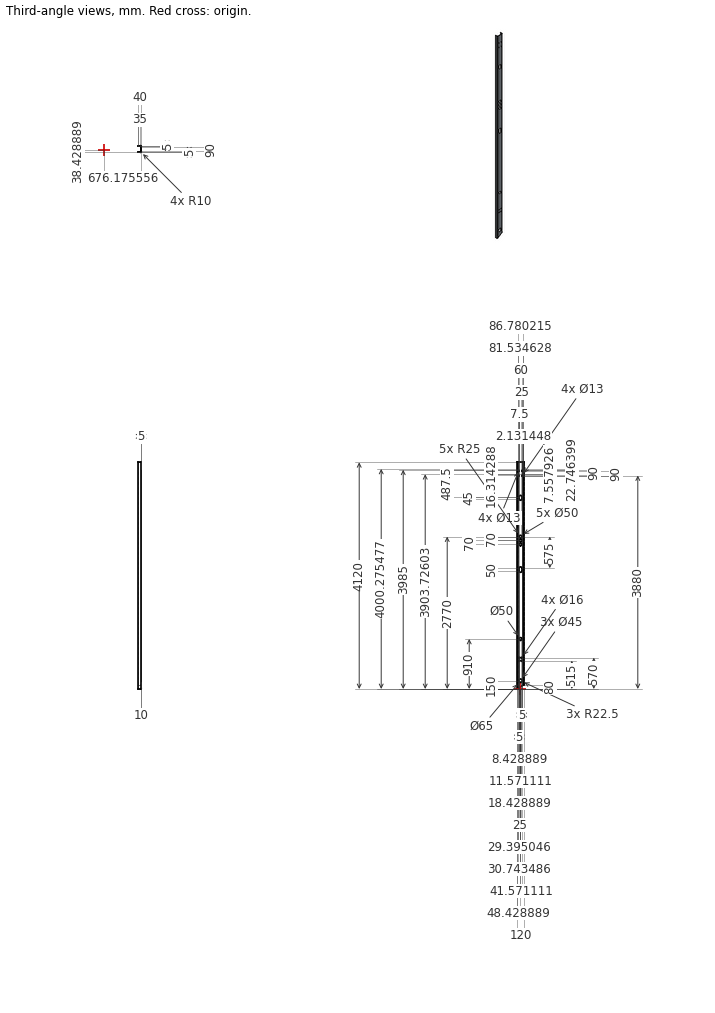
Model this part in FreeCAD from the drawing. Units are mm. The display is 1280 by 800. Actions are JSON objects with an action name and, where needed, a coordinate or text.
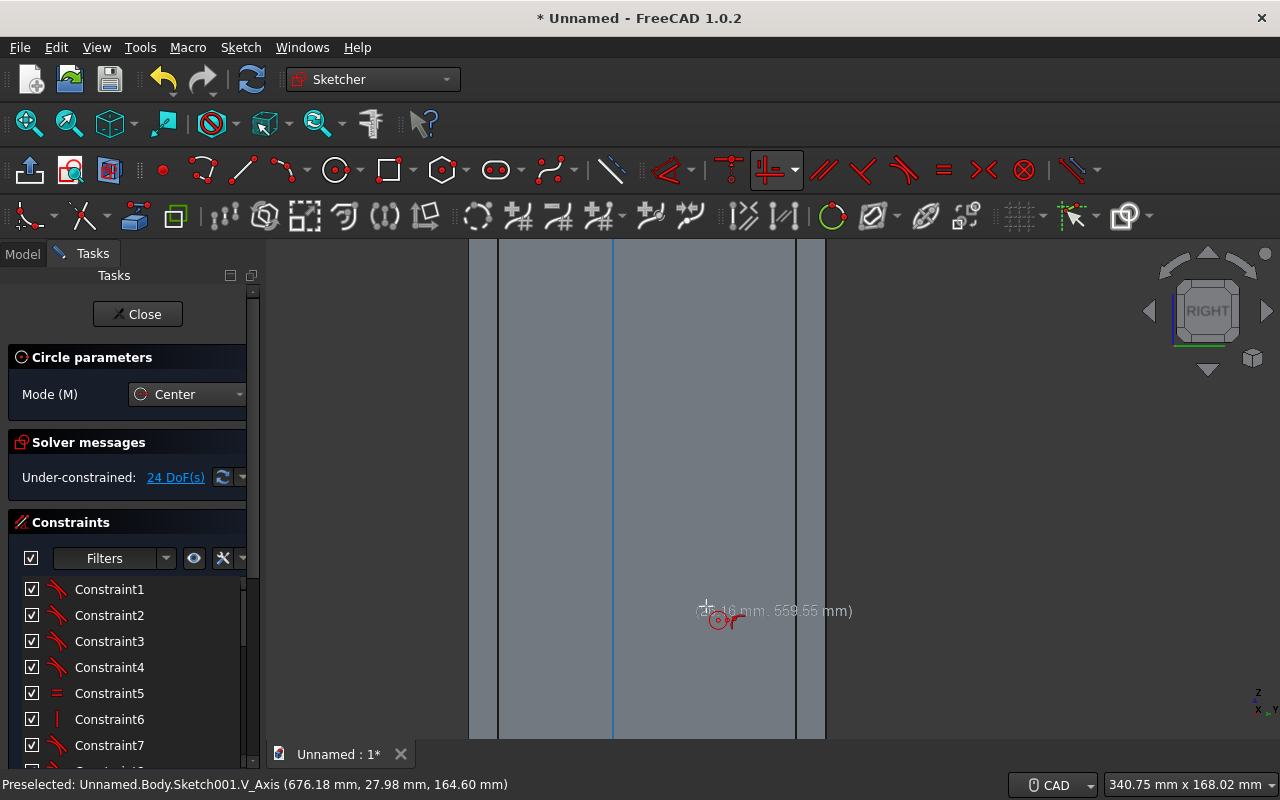
{"action": "scroll", "coordinate": [706, 605], "scroll_direction": "down", "scroll_amount": 18}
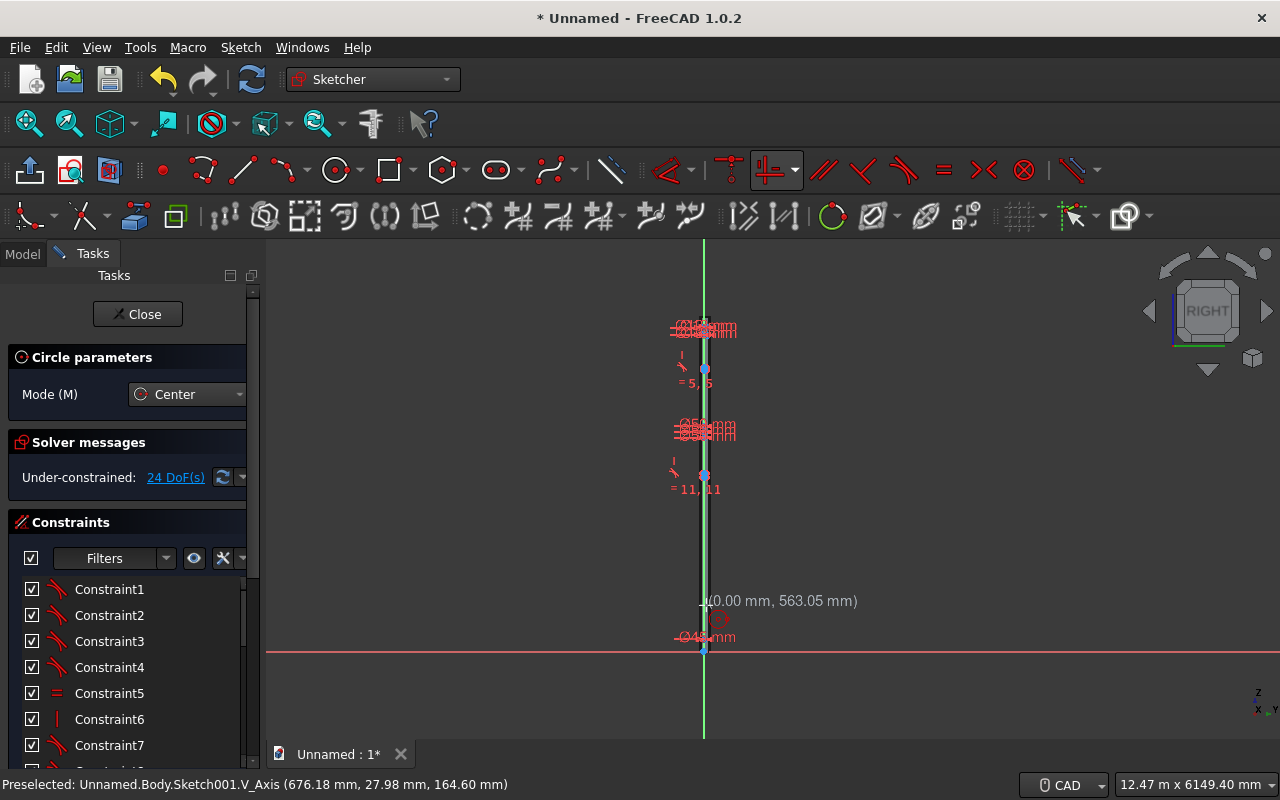
{"action": "scroll", "coordinate": [706, 605], "scroll_direction": "up", "scroll_amount": 10}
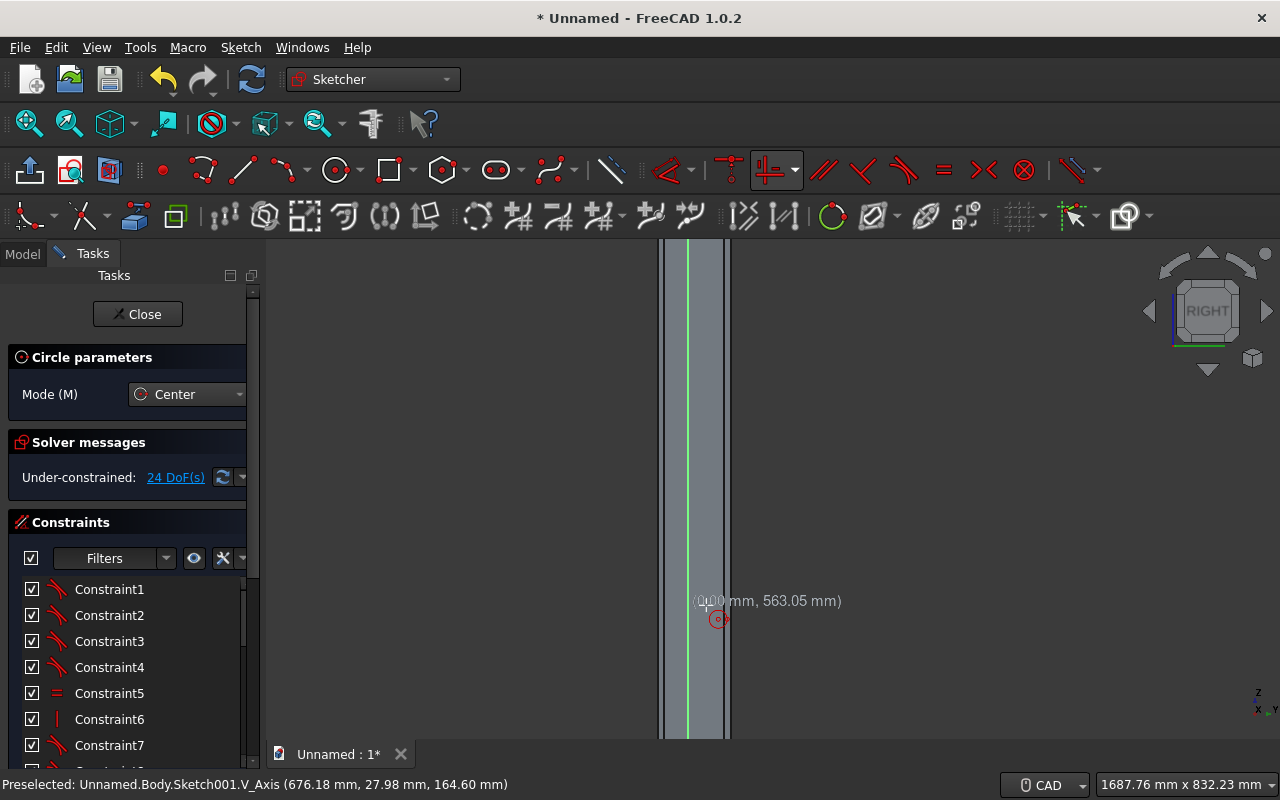
{"action": "left_click", "coordinate": [706, 602]}
{"action": "mouse_move", "coordinate": [710, 598]}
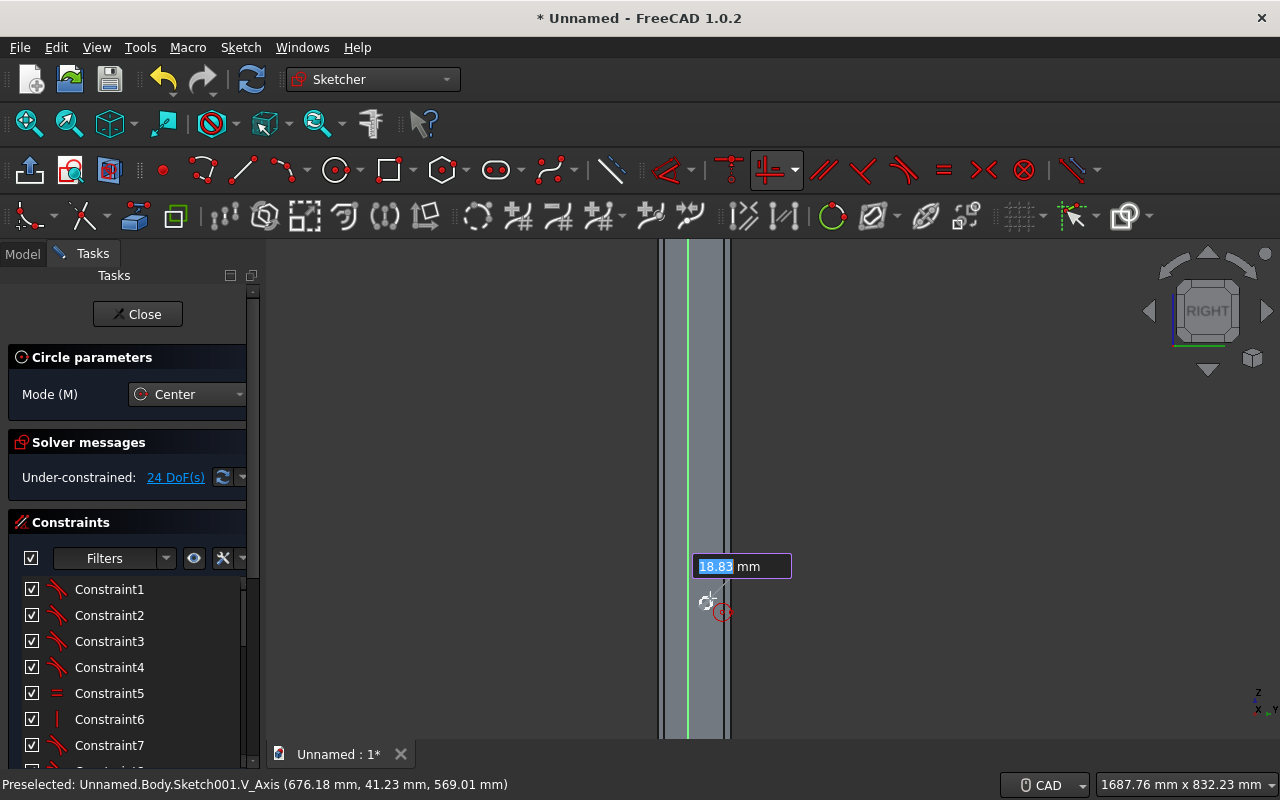
{"action": "type", "text": "16"}
{"action": "key", "text": "Return"}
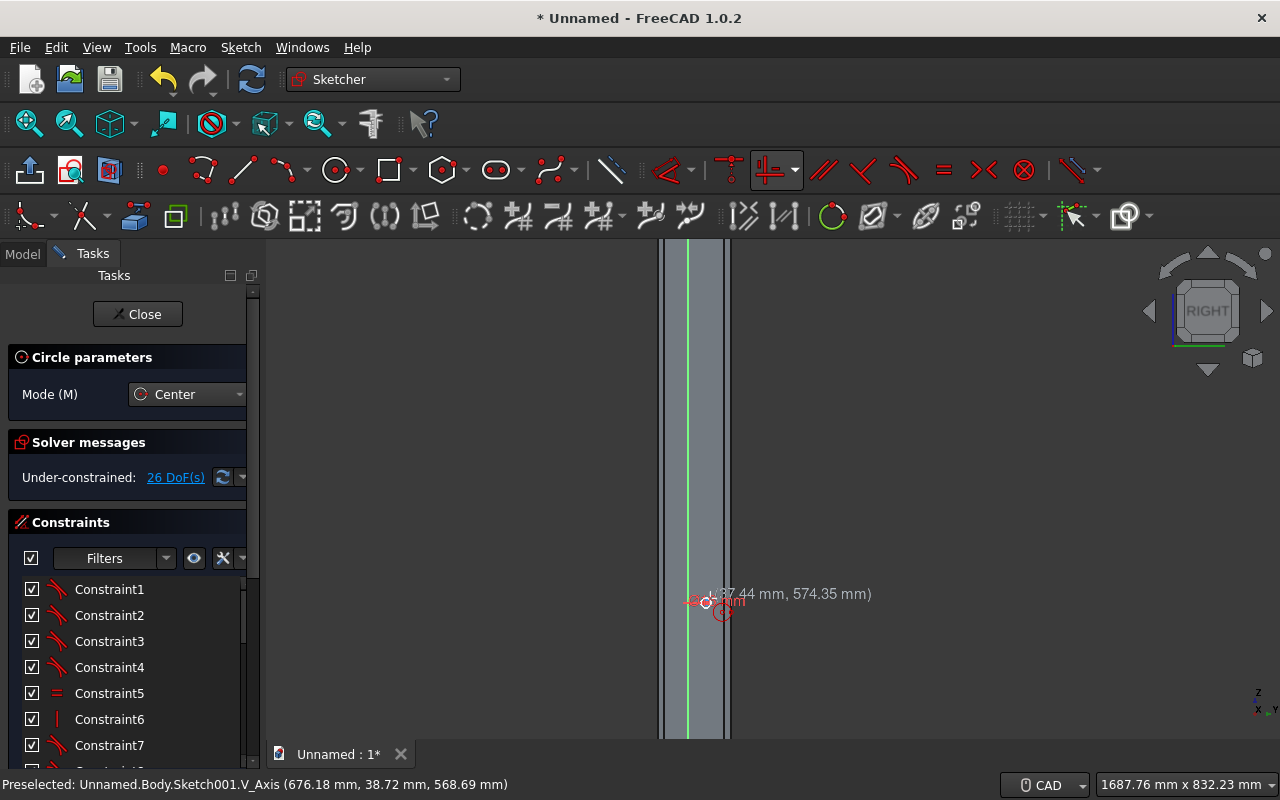
{"action": "scroll", "coordinate": [706, 635], "scroll_direction": "up", "scroll_amount": 8}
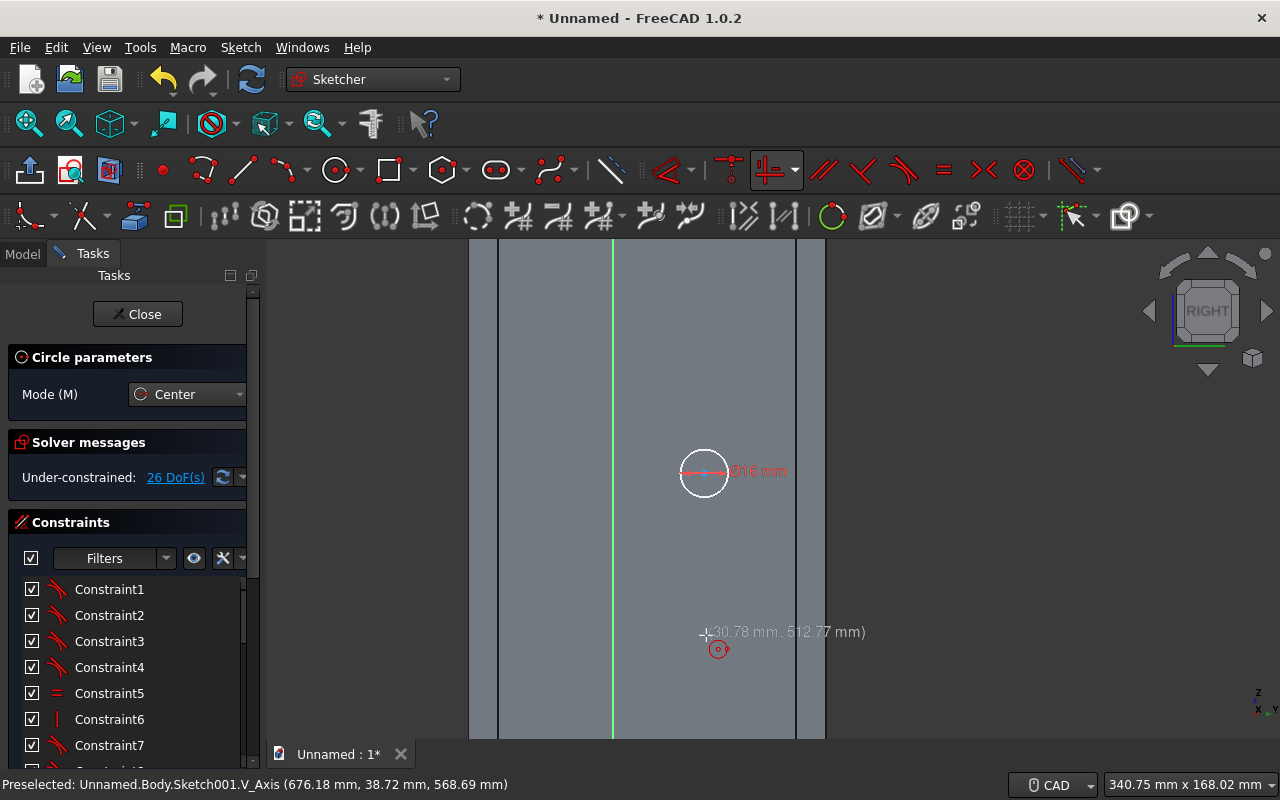
{"action": "scroll", "coordinate": [706, 609], "scroll_direction": "down", "scroll_amount": 18}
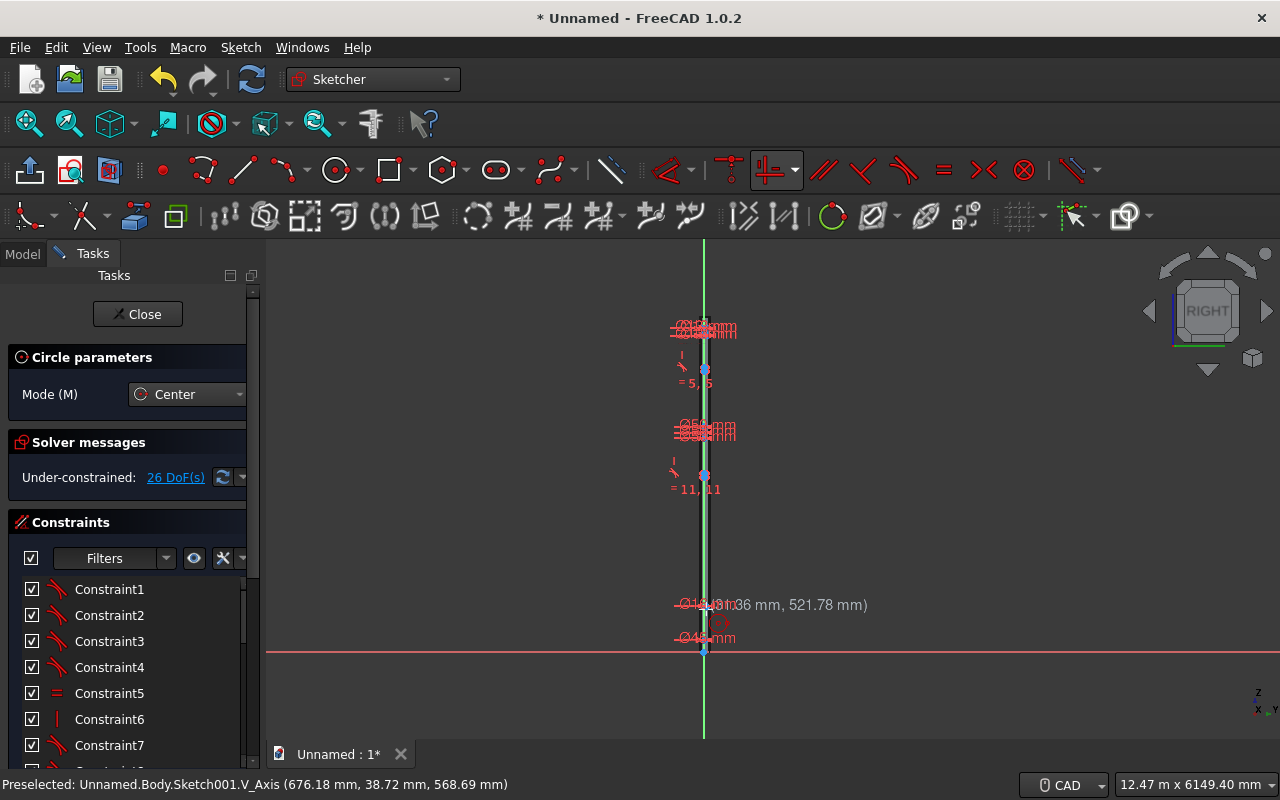
{"action": "scroll", "coordinate": [706, 610], "scroll_direction": "up", "scroll_amount": 10}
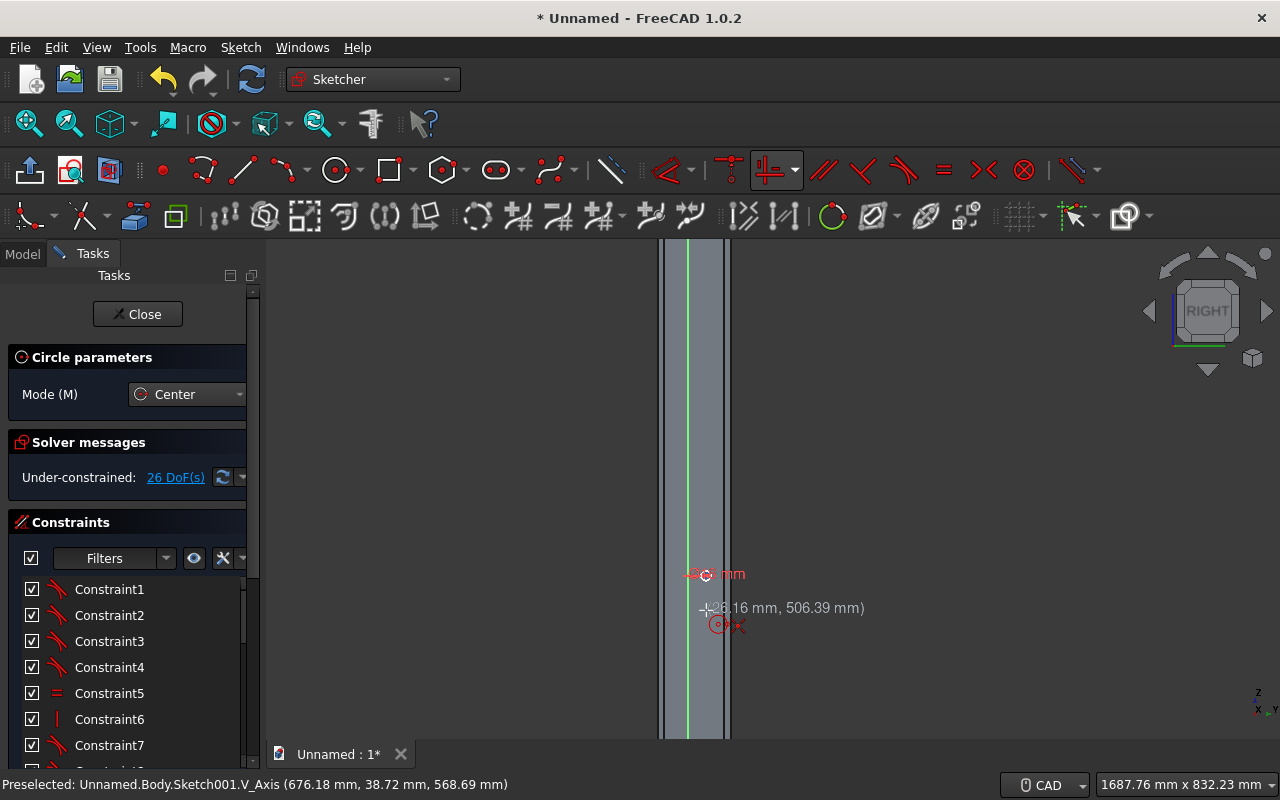
{"action": "left_click", "coordinate": [706, 607]}
{"action": "mouse_move", "coordinate": [710, 604]}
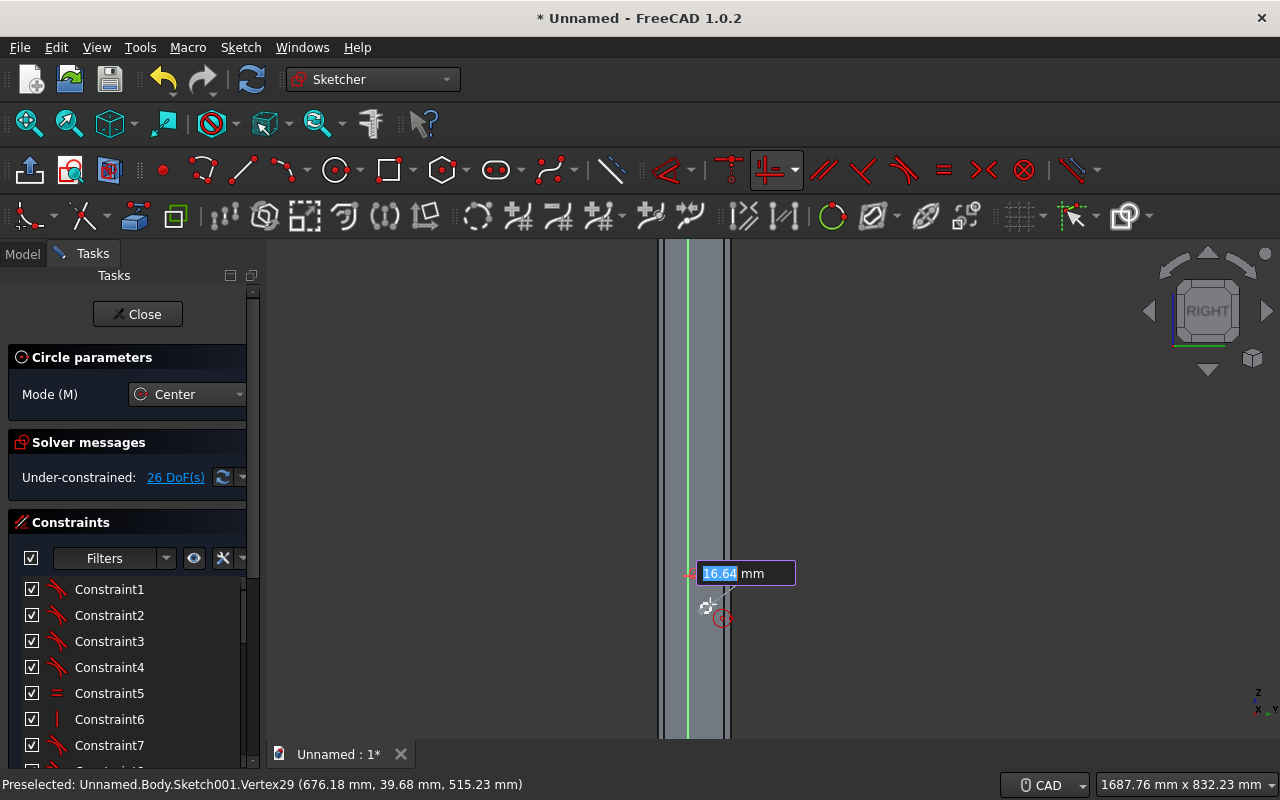
{"action": "type", "text": "16"}
{"action": "key", "text": "Return"}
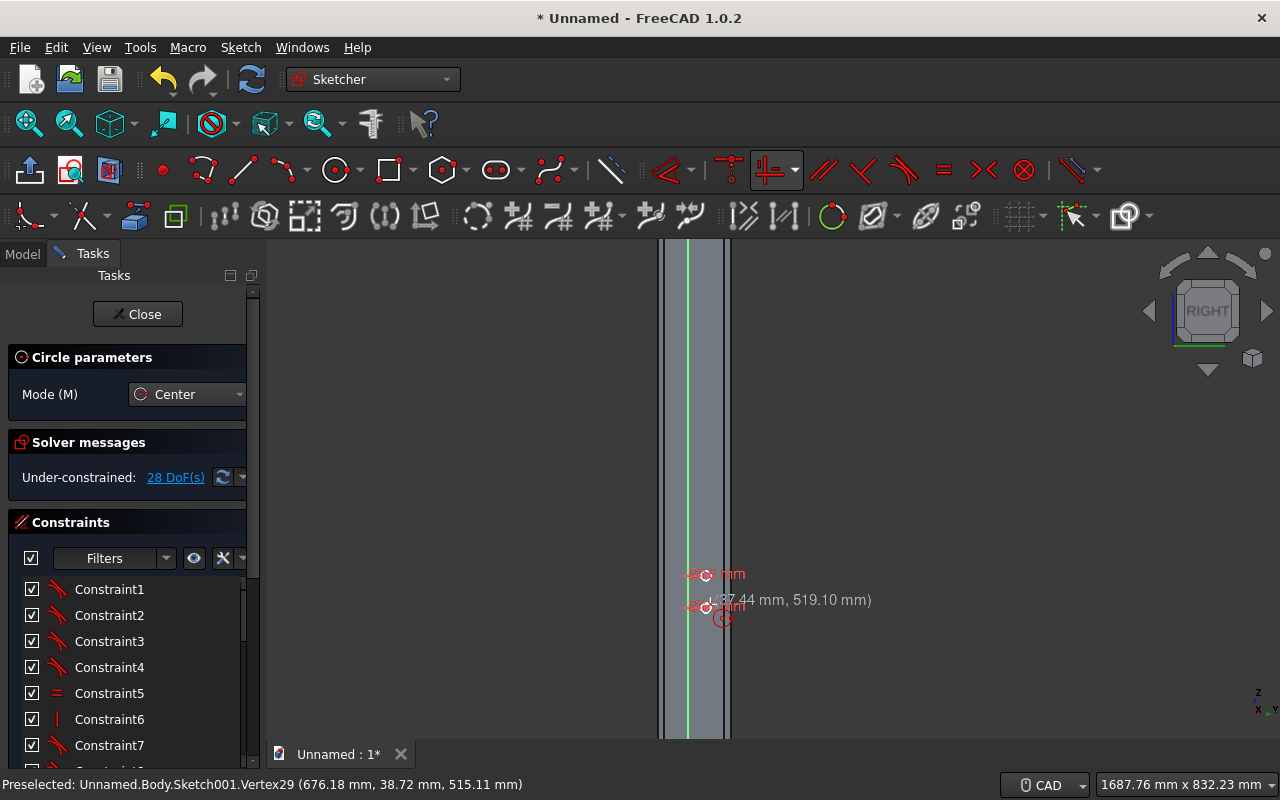
{"action": "scroll", "coordinate": [682, 574], "scroll_direction": "up", "scroll_amount": 8}